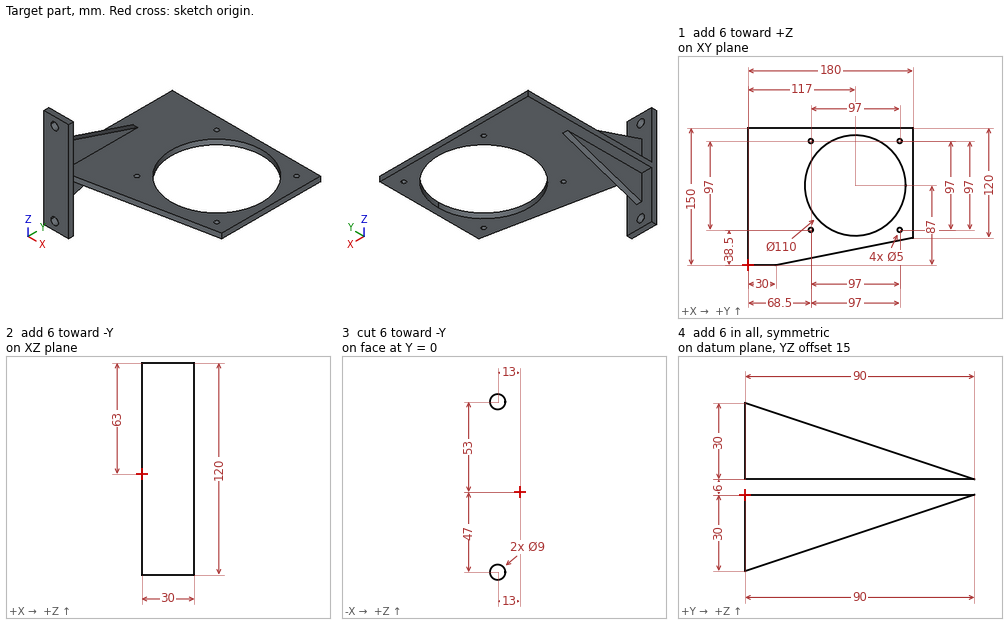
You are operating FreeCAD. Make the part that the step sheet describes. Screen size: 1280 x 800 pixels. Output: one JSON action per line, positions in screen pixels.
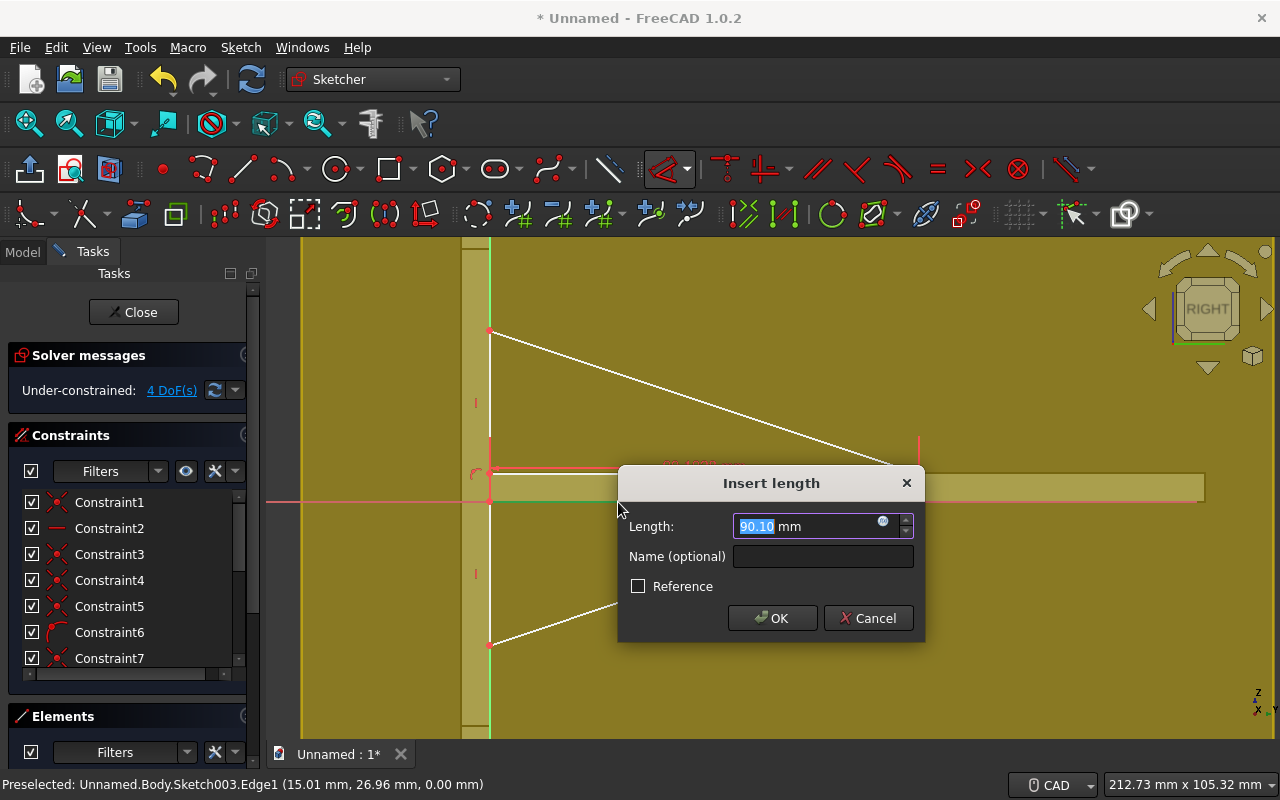
{"action": "type", "text": "90"}
{"action": "key", "text": "Return"}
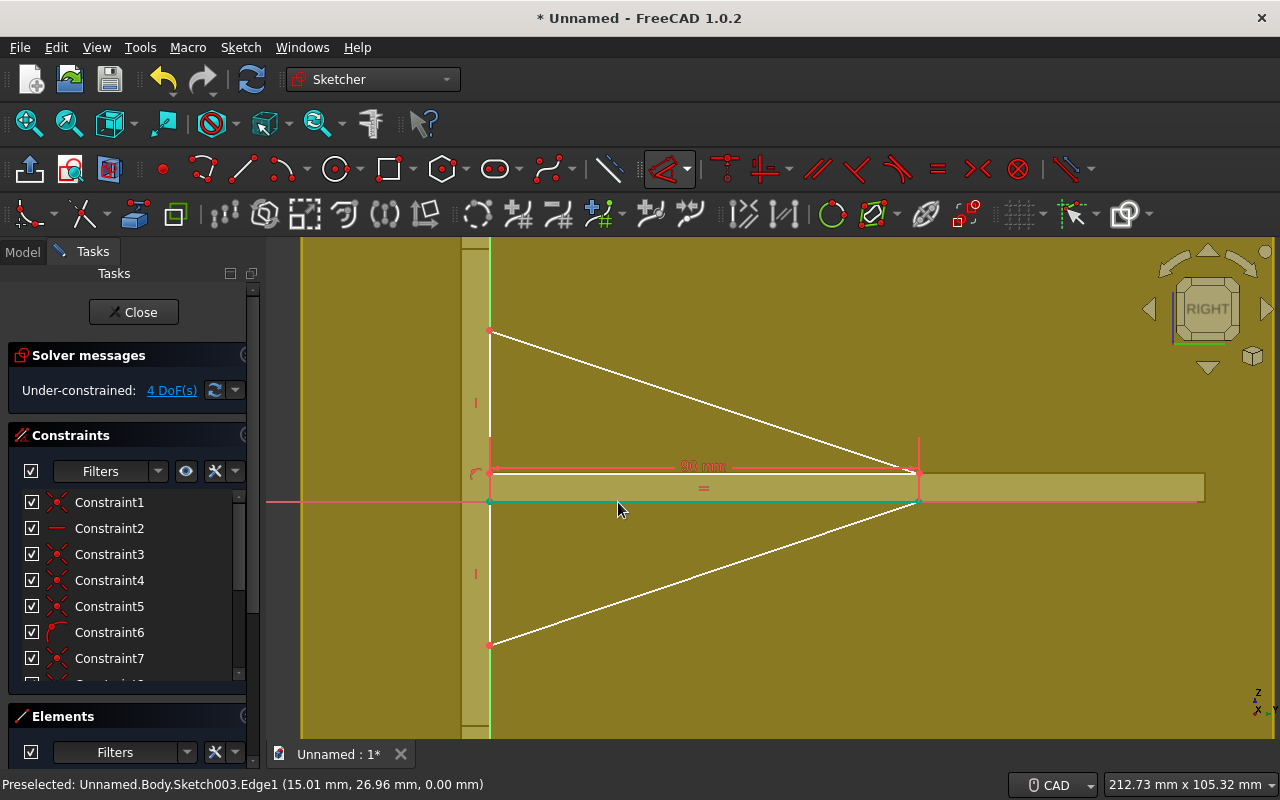
{"action": "left_click", "coordinate": [490, 603]}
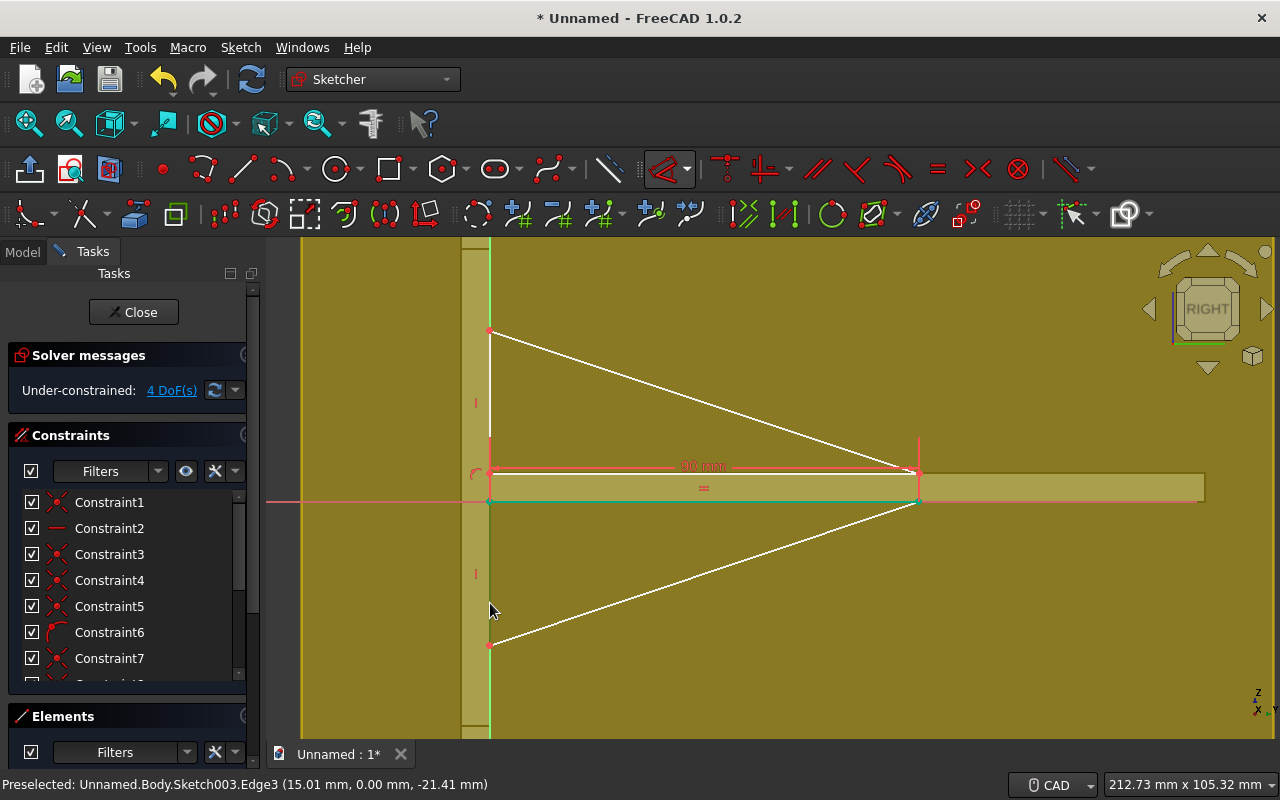
{"action": "key", "text": "i"}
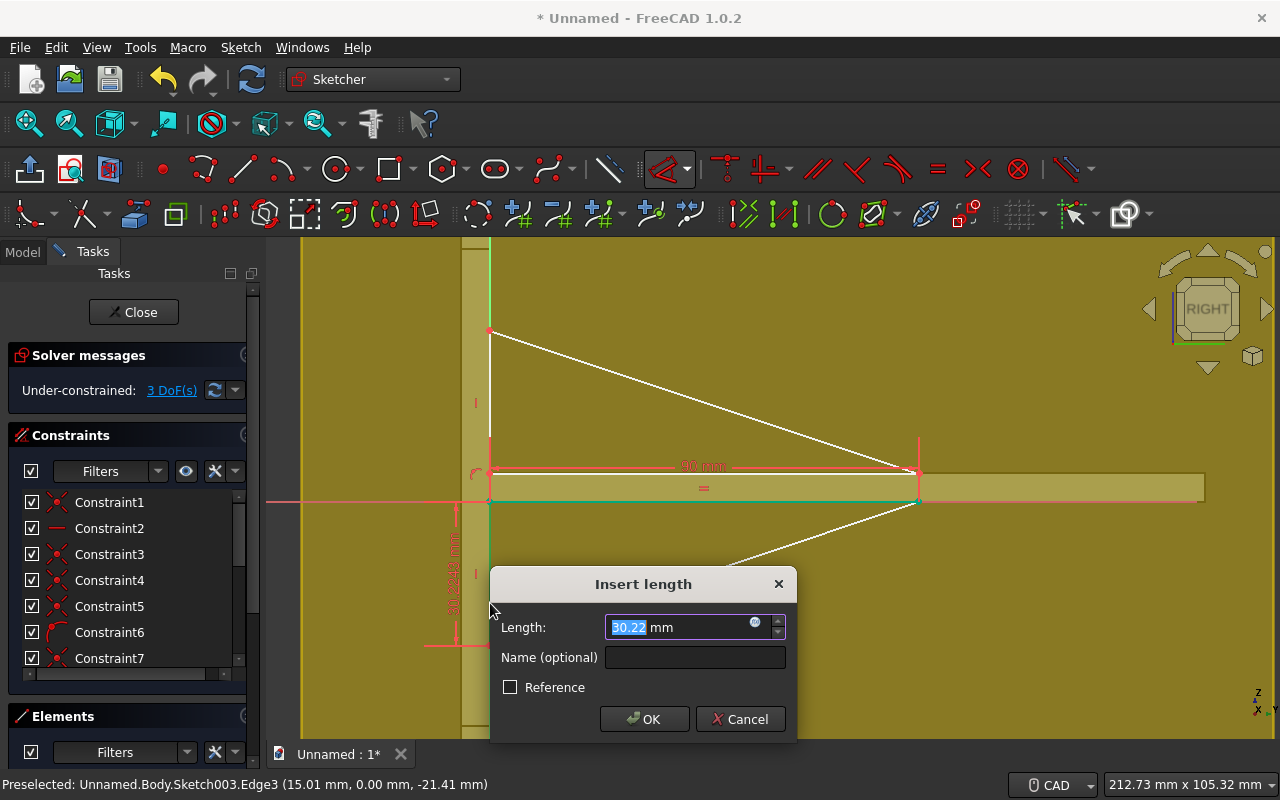
{"action": "type", "text": "30"}
{"action": "key", "text": "Return"}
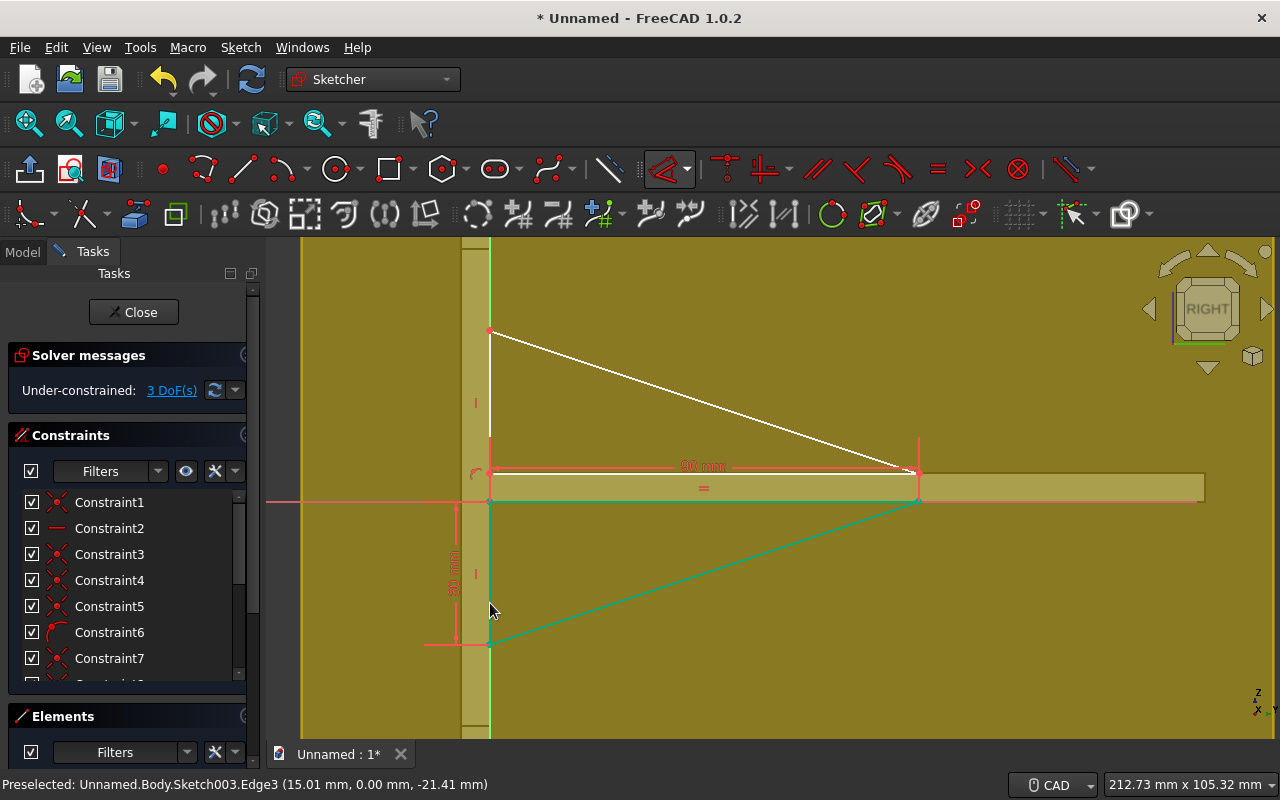
{"action": "left_click", "coordinate": [490, 431]}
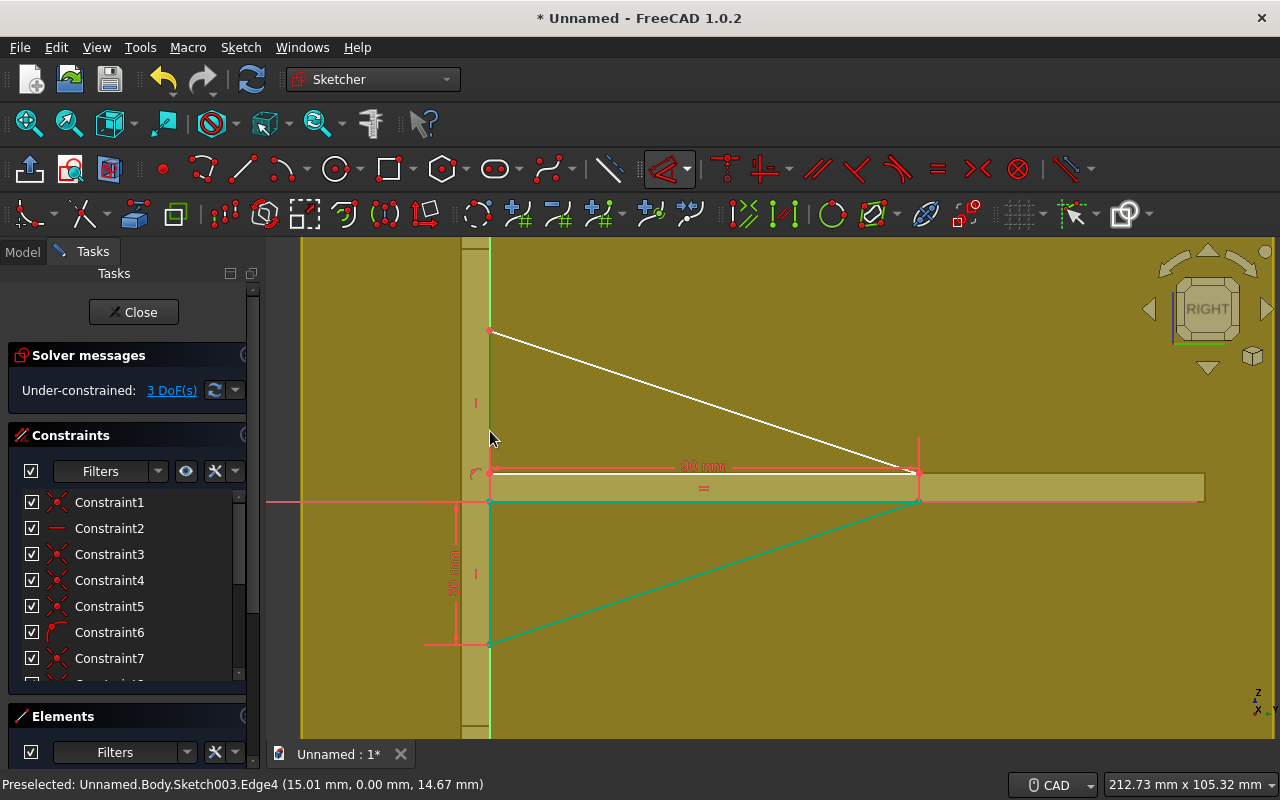
{"action": "key", "text": "i"}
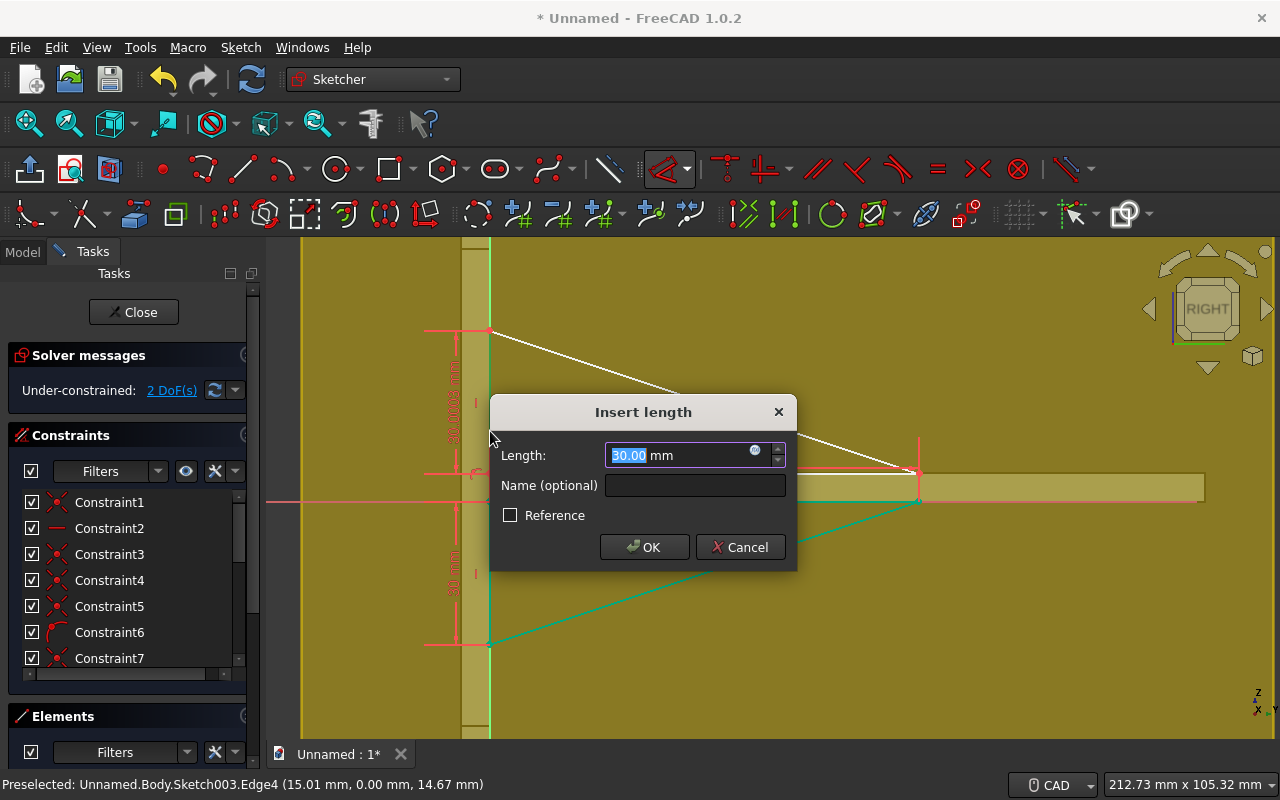
{"action": "type", "text": "30"}
{"action": "key", "text": "Return"}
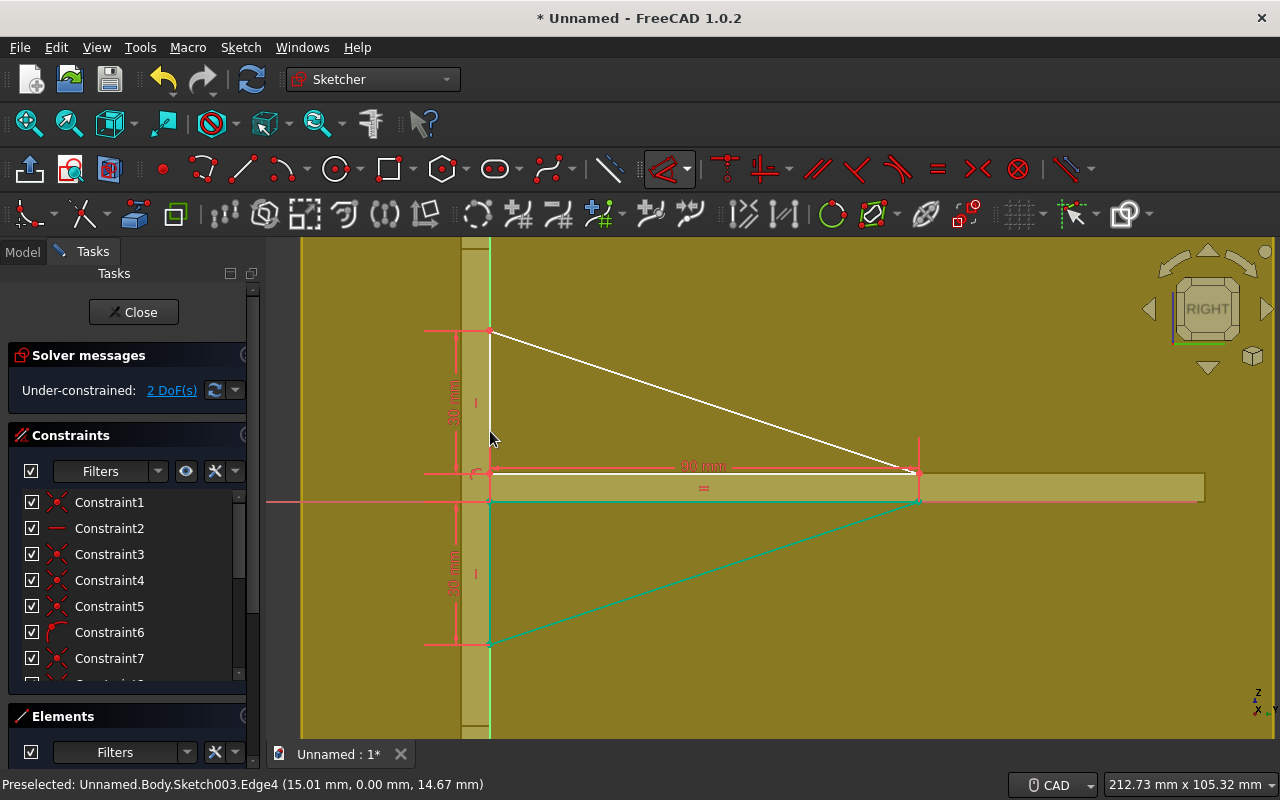
{"action": "left_click", "coordinate": [790, 474]}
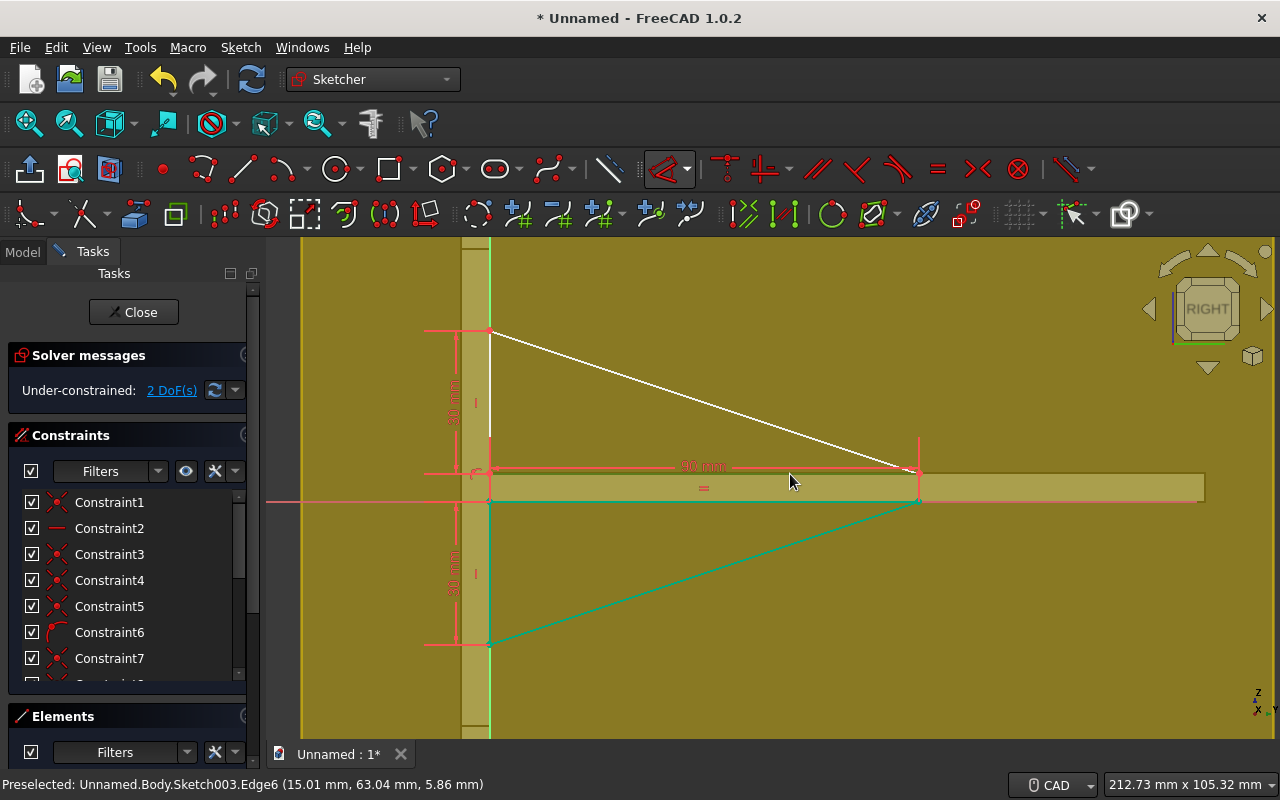
{"action": "key", "text": "l"}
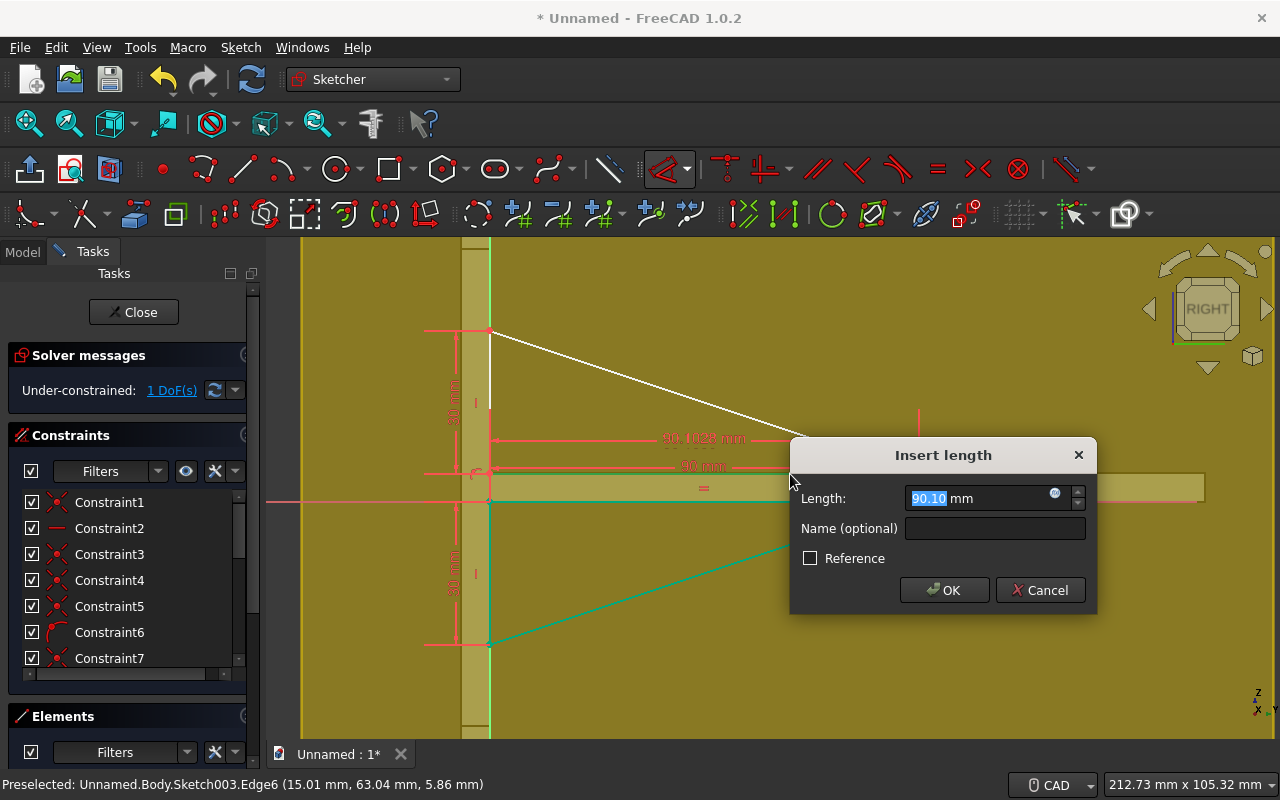
{"action": "type", "text": "90"}
{"action": "key", "text": "Return"}